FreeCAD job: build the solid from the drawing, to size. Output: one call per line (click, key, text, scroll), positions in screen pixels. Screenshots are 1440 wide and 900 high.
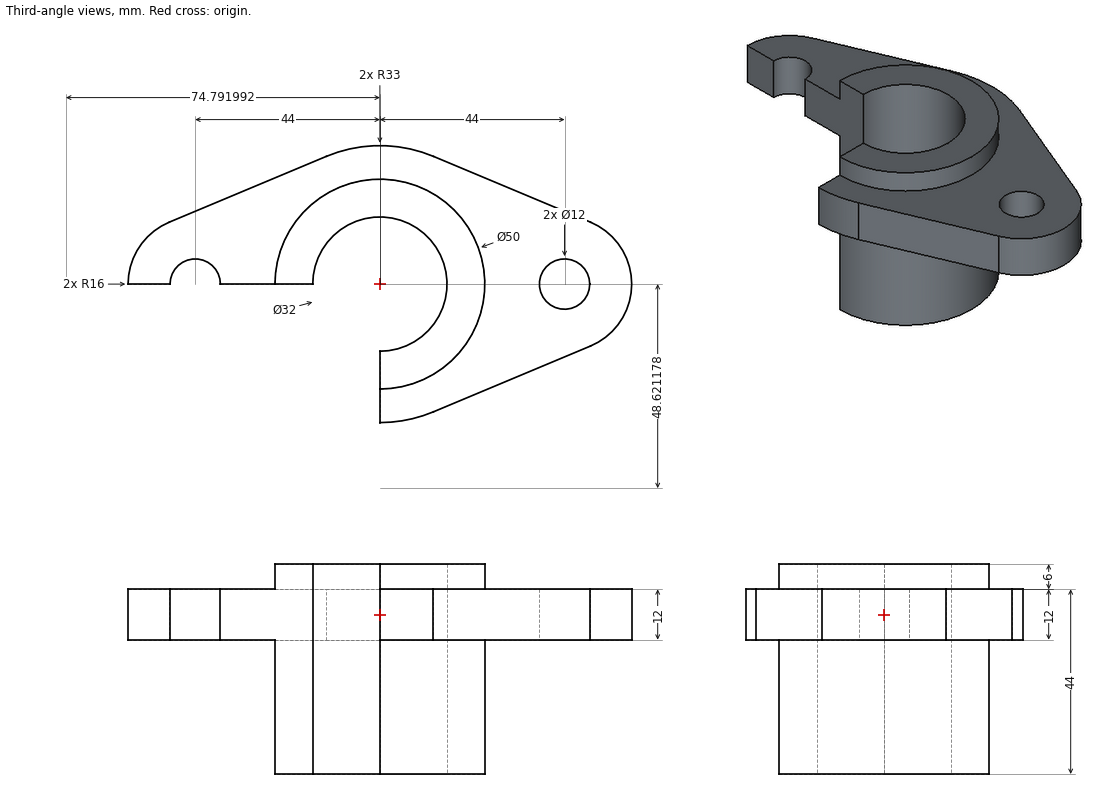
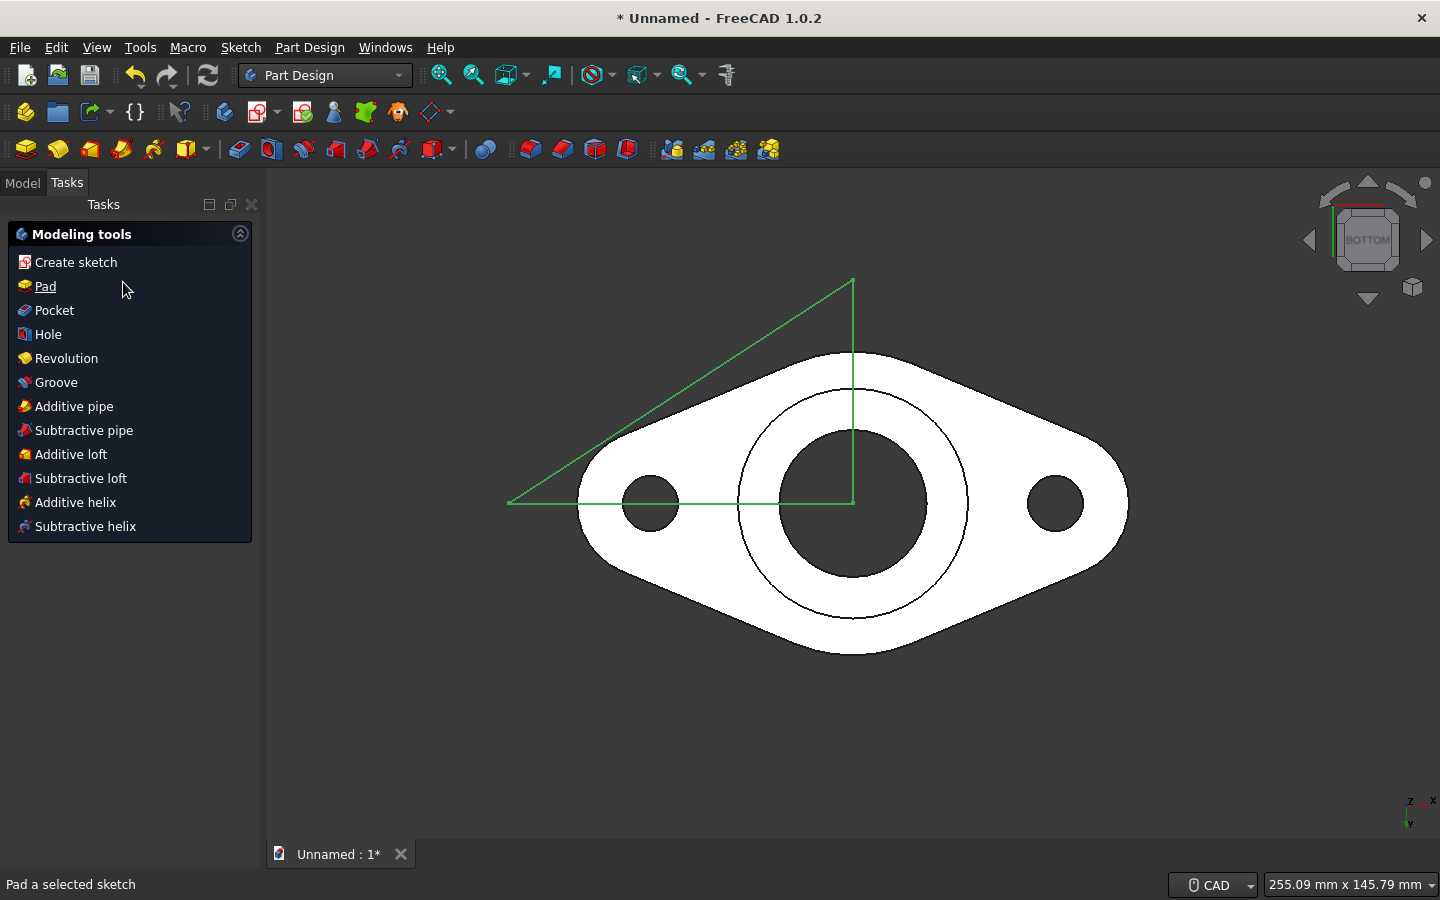
click(240, 150)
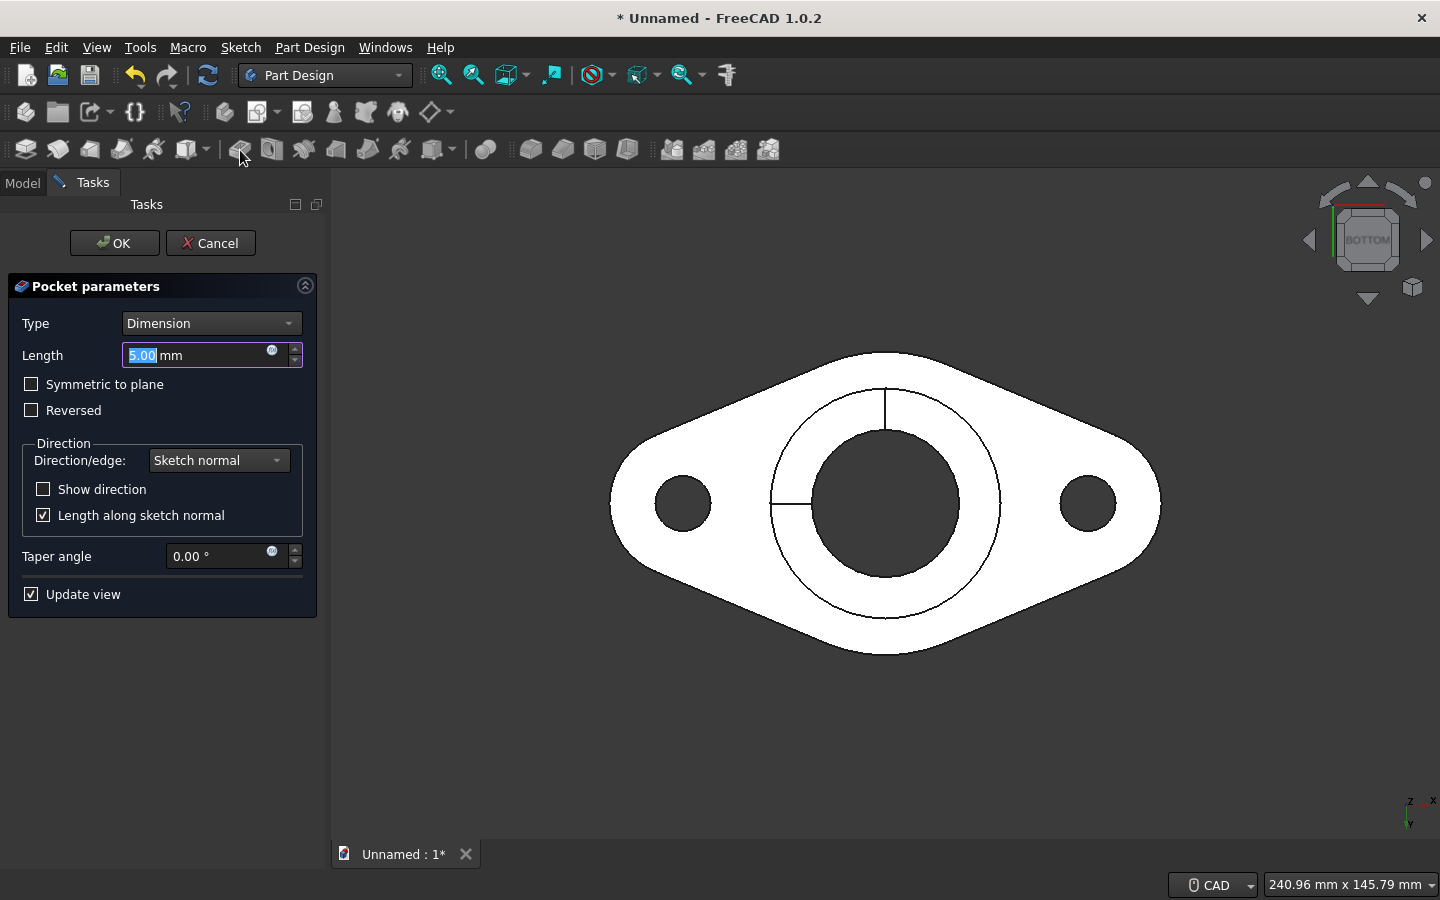
click(212, 324)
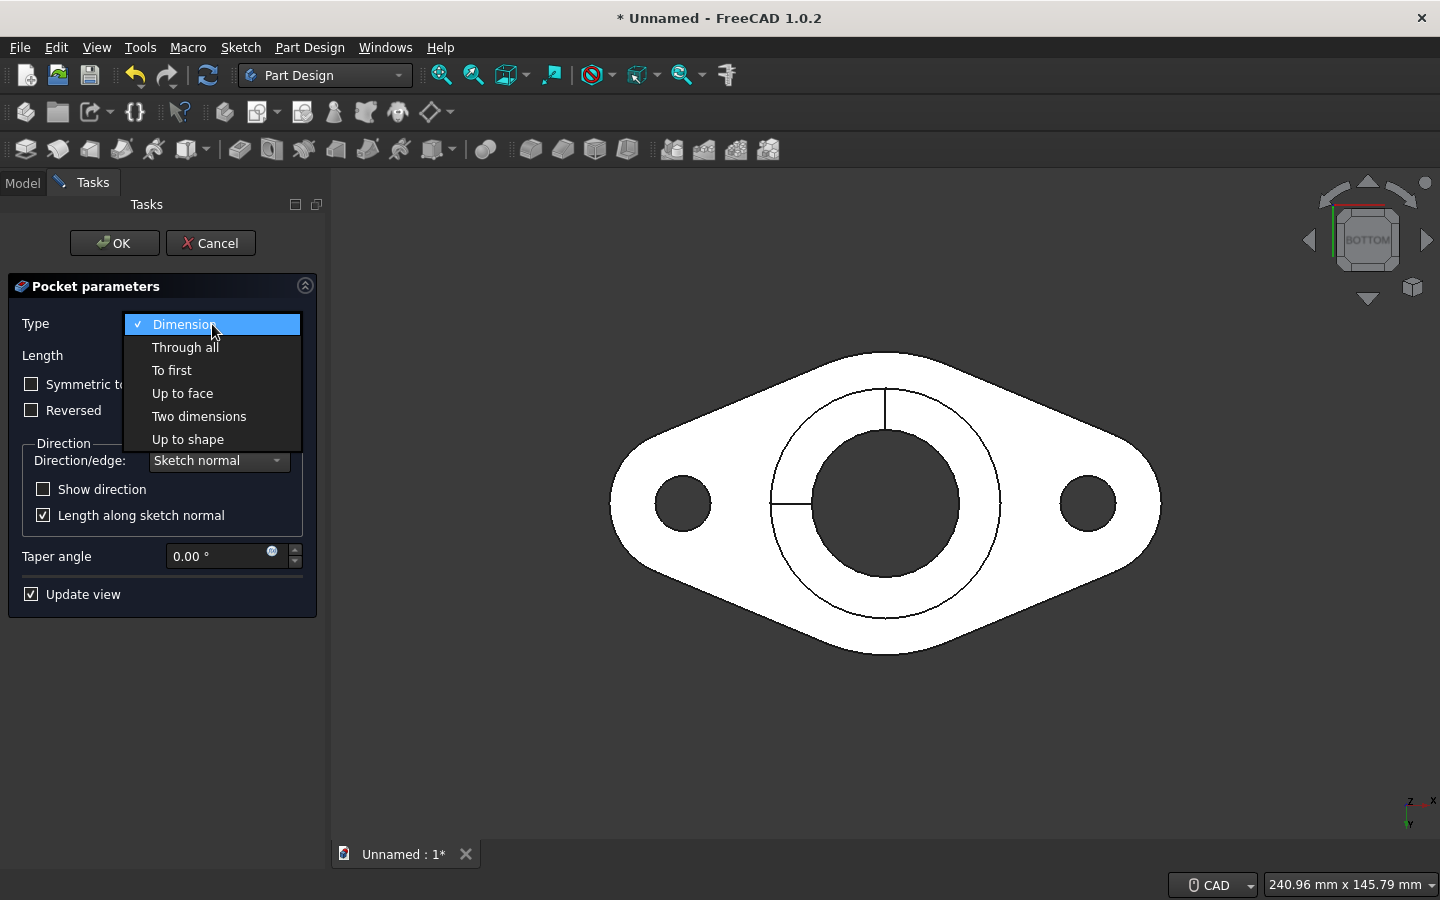
click(212, 348)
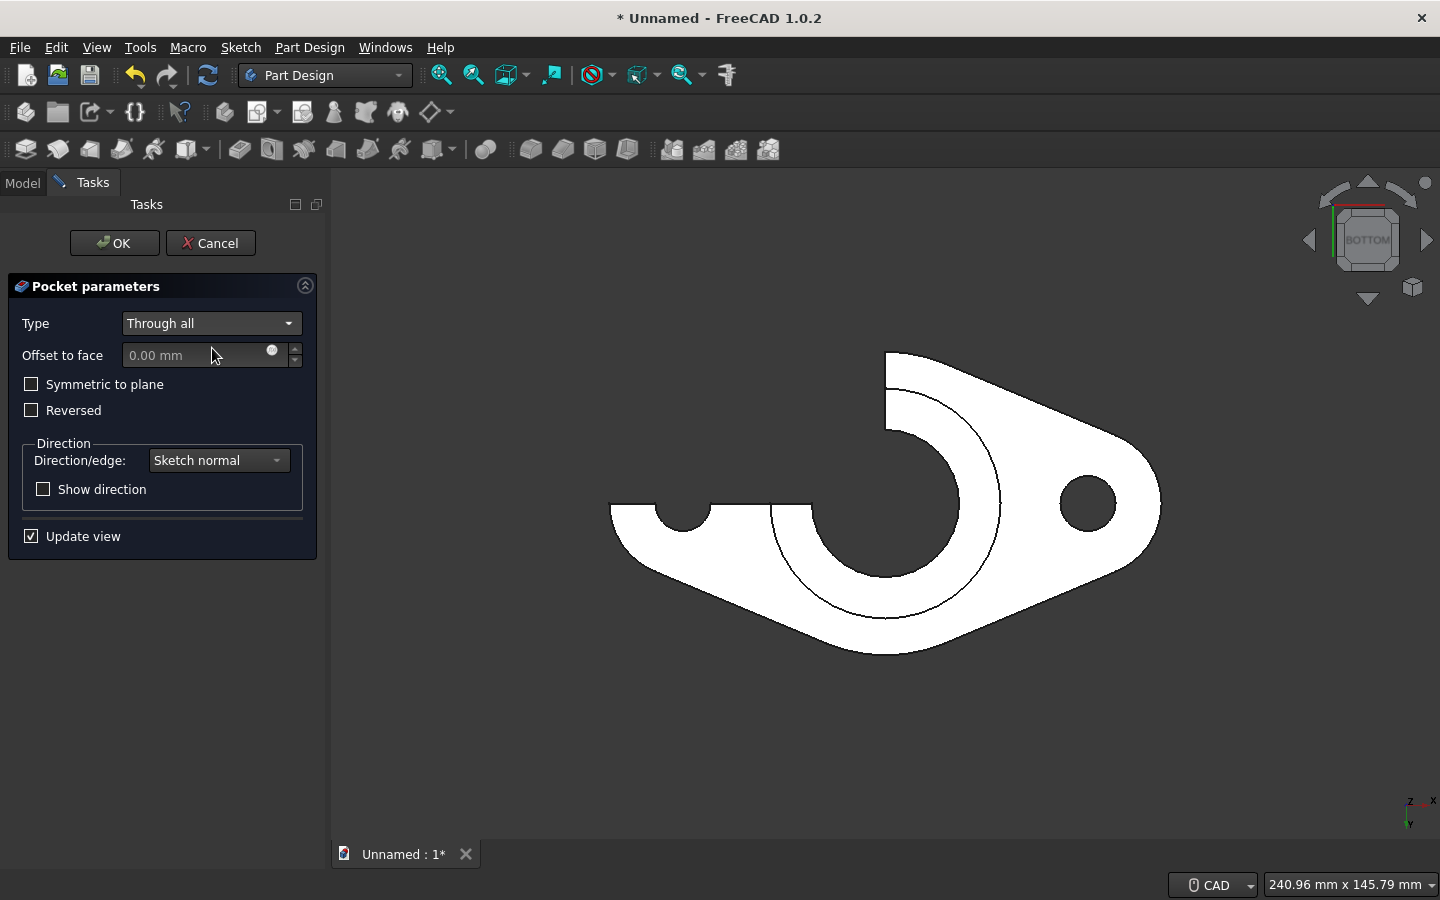
click(115, 243)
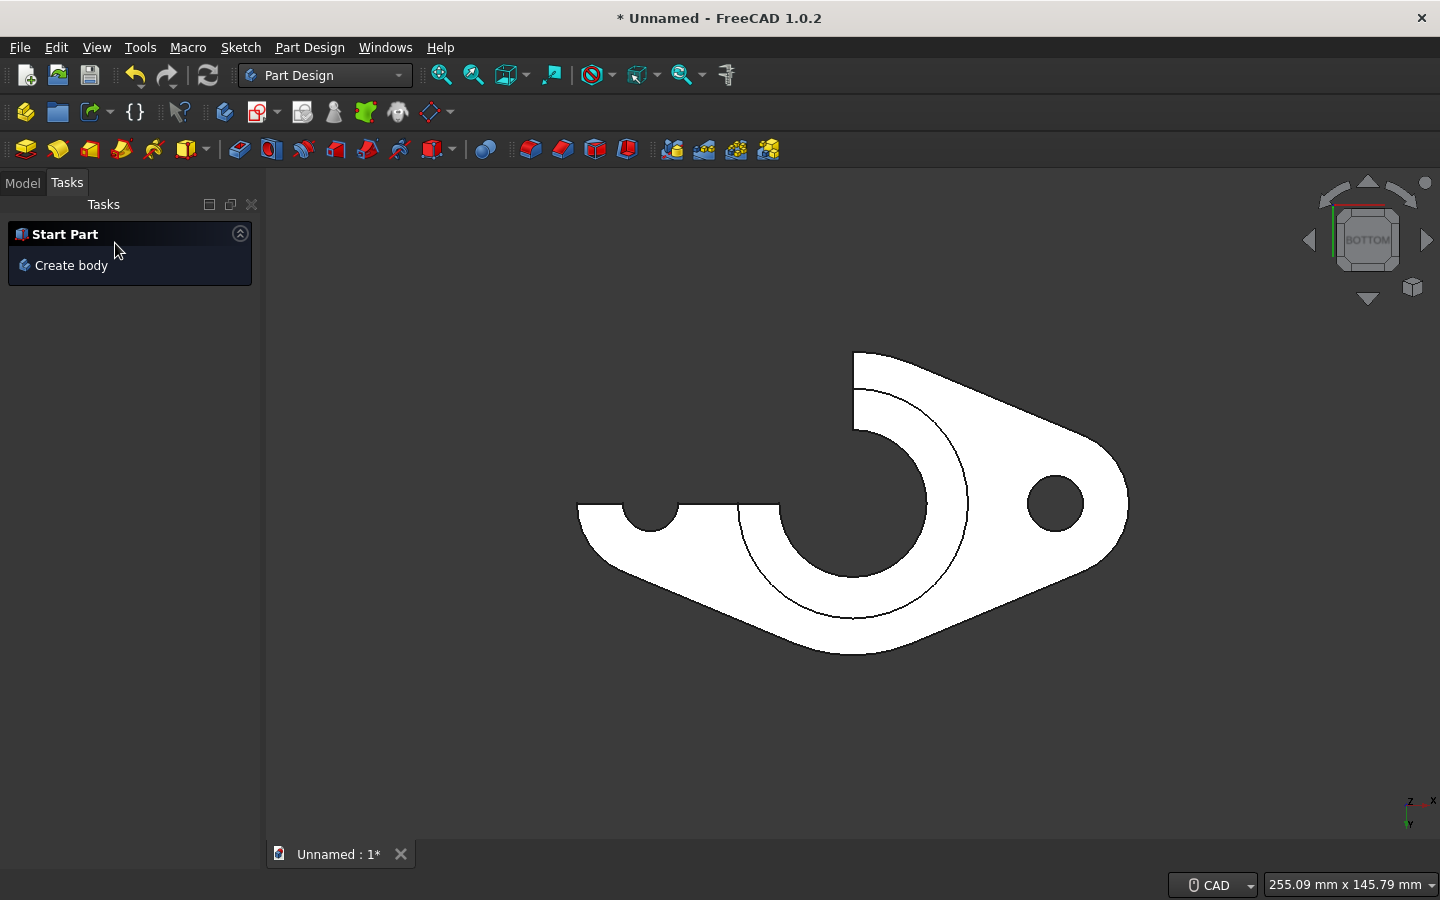
key(0)